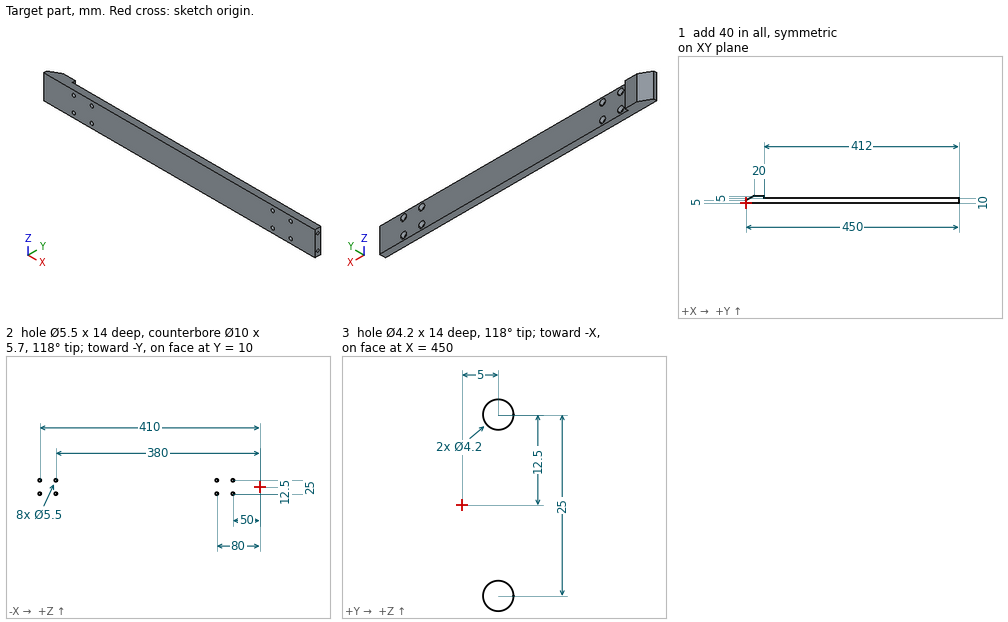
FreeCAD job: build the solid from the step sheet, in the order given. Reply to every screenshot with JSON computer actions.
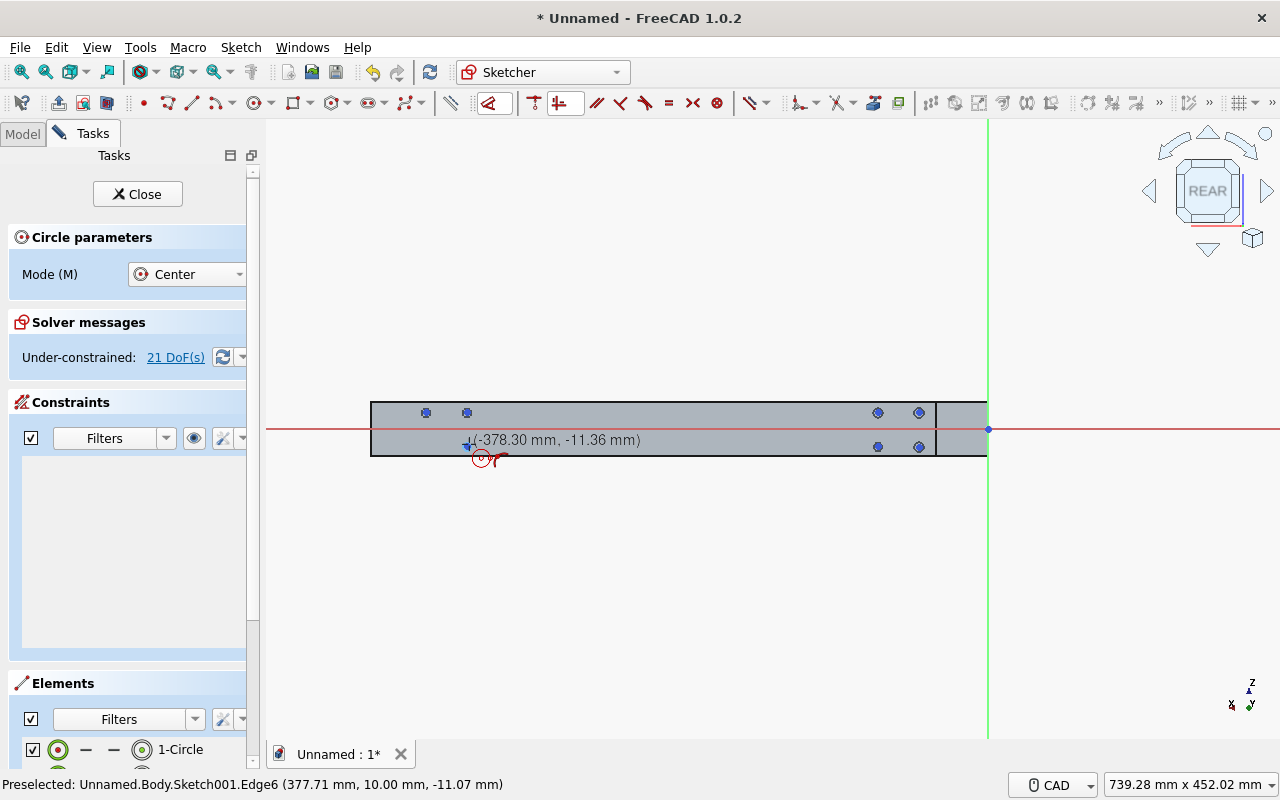
{"action": "scroll", "coordinate": [426, 446], "scroll_direction": "up", "scroll_amount": 9}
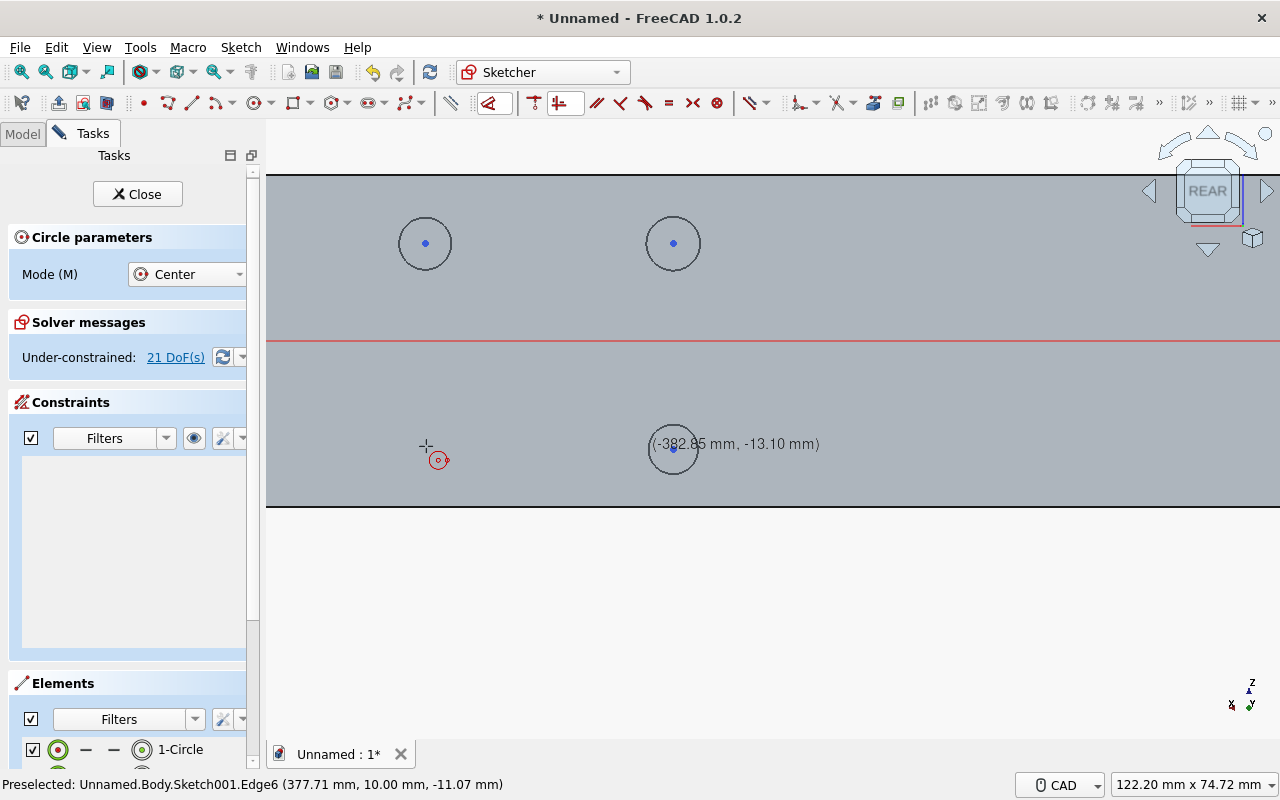
{"action": "scroll", "coordinate": [426, 446], "scroll_direction": "down", "scroll_amount": 9}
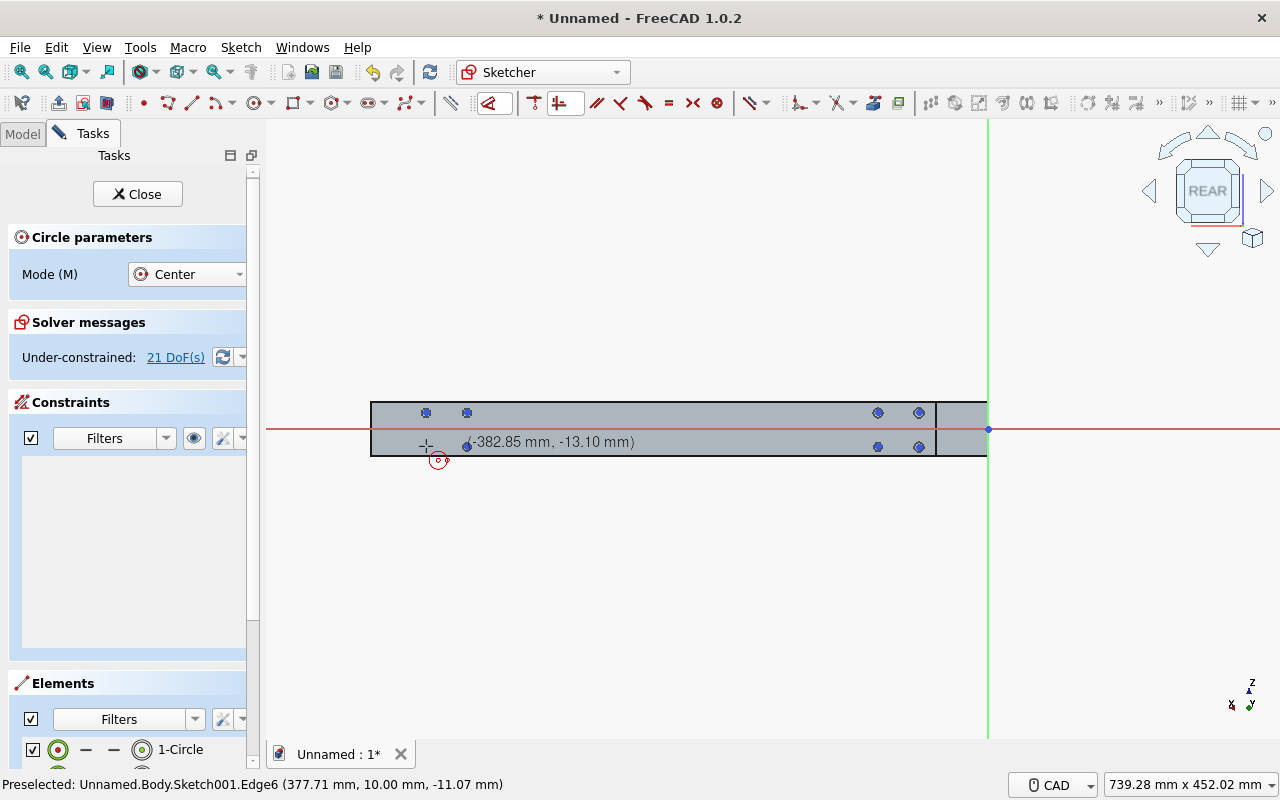
{"action": "left_click", "coordinate": [426, 446]}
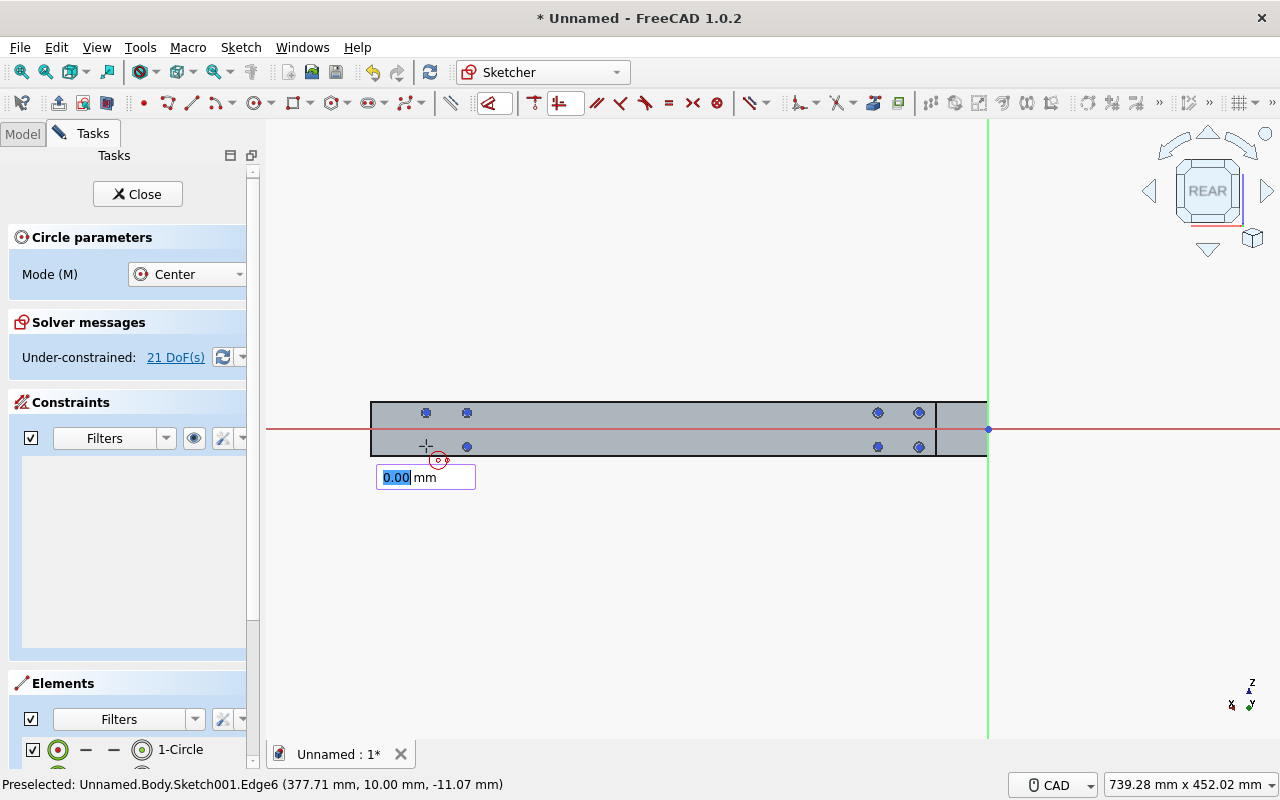
{"action": "scroll", "coordinate": [428, 444], "scroll_direction": "up", "scroll_amount": 8}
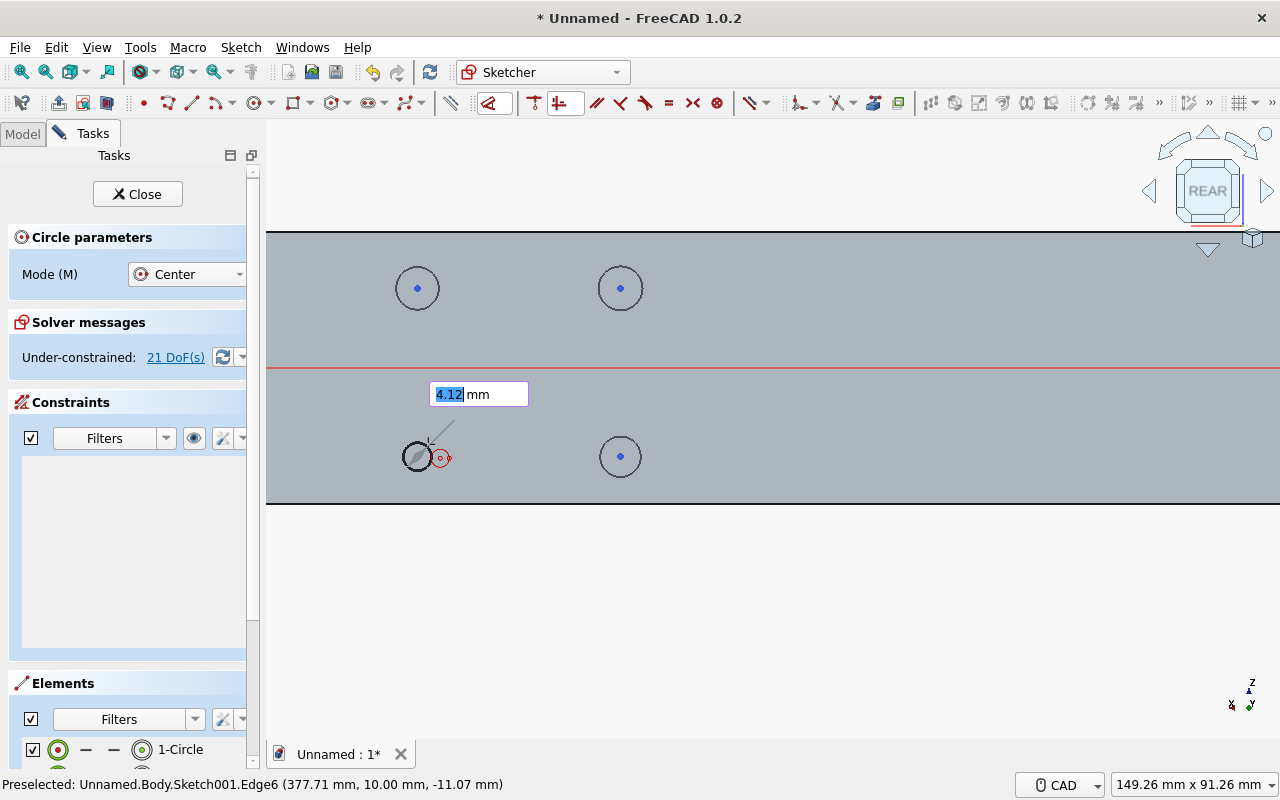
{"action": "left_click", "coordinate": [429, 440]}
{"action": "key", "text": "Escape"}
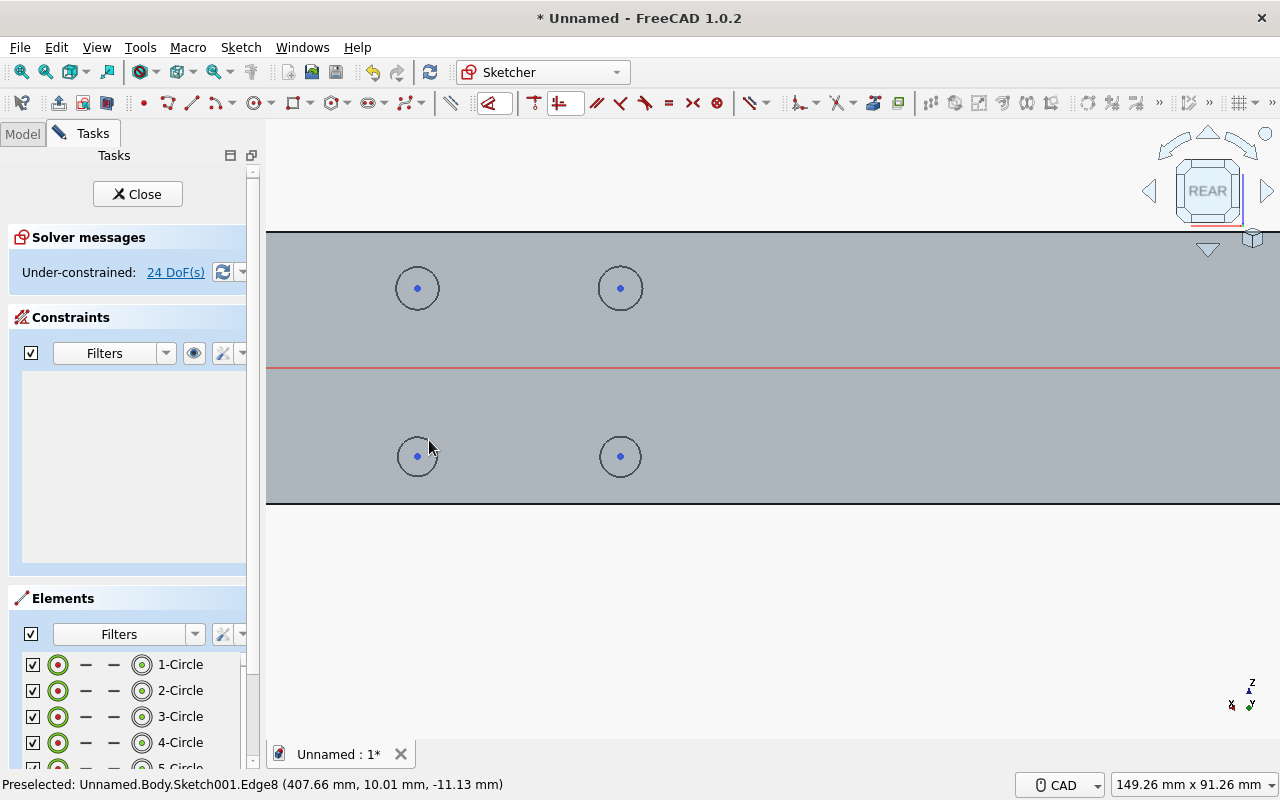
{"action": "scroll", "coordinate": [428, 444], "scroll_direction": "down", "scroll_amount": 8}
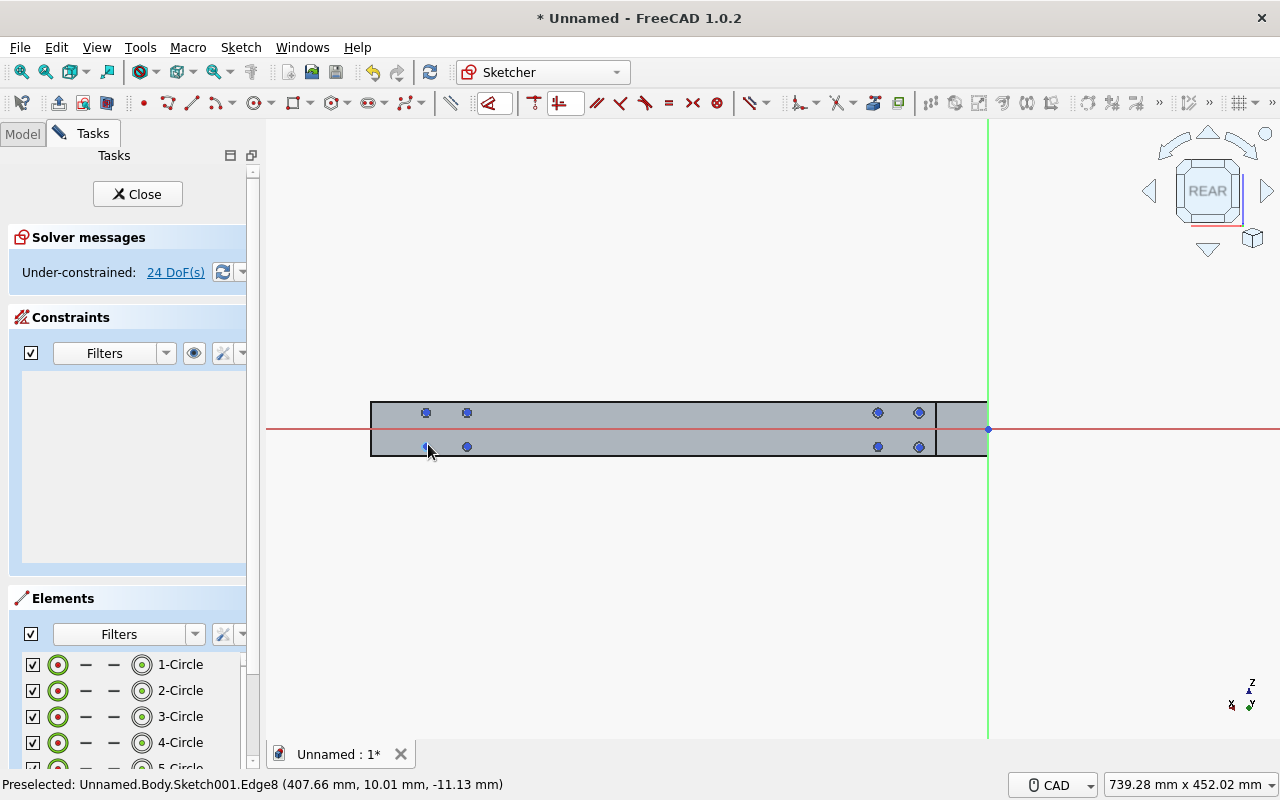
{"action": "scroll", "coordinate": [922, 444], "scroll_direction": "up", "scroll_amount": 6}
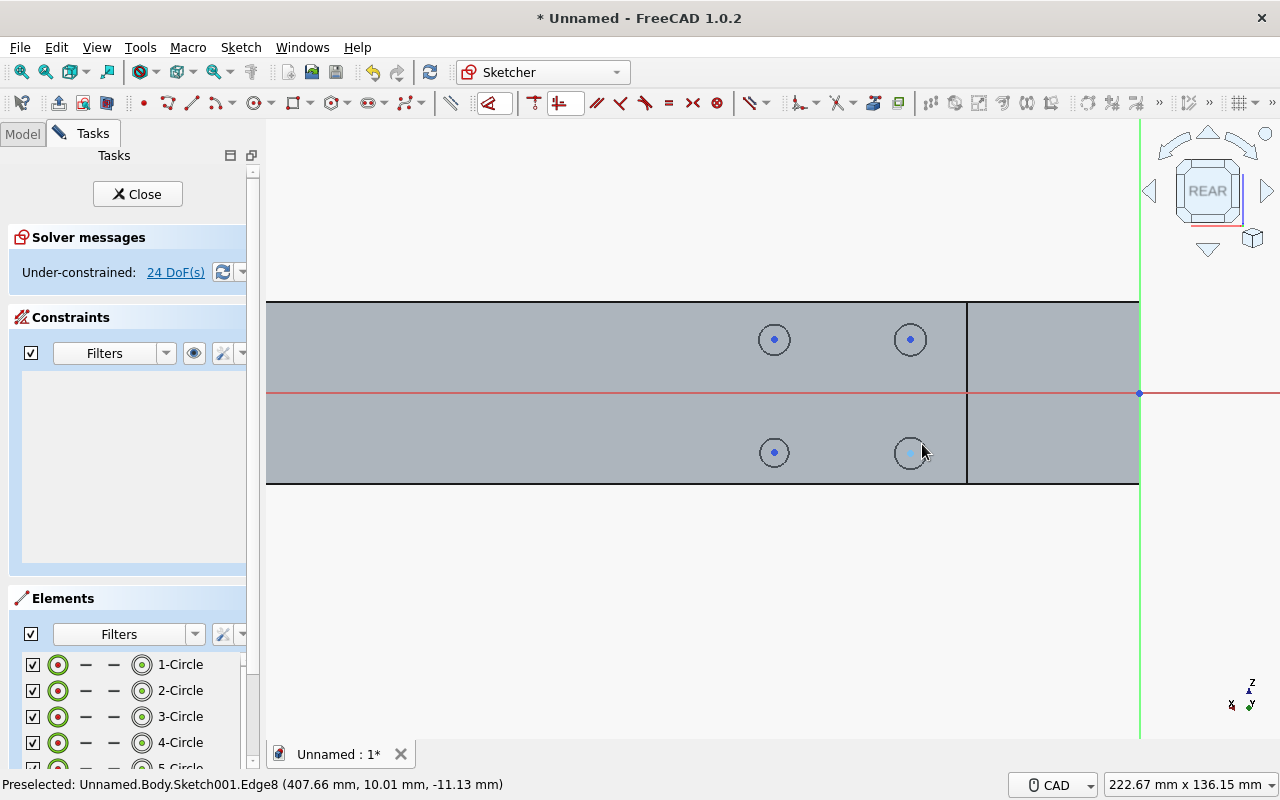
{"action": "left_click", "coordinate": [922, 442]}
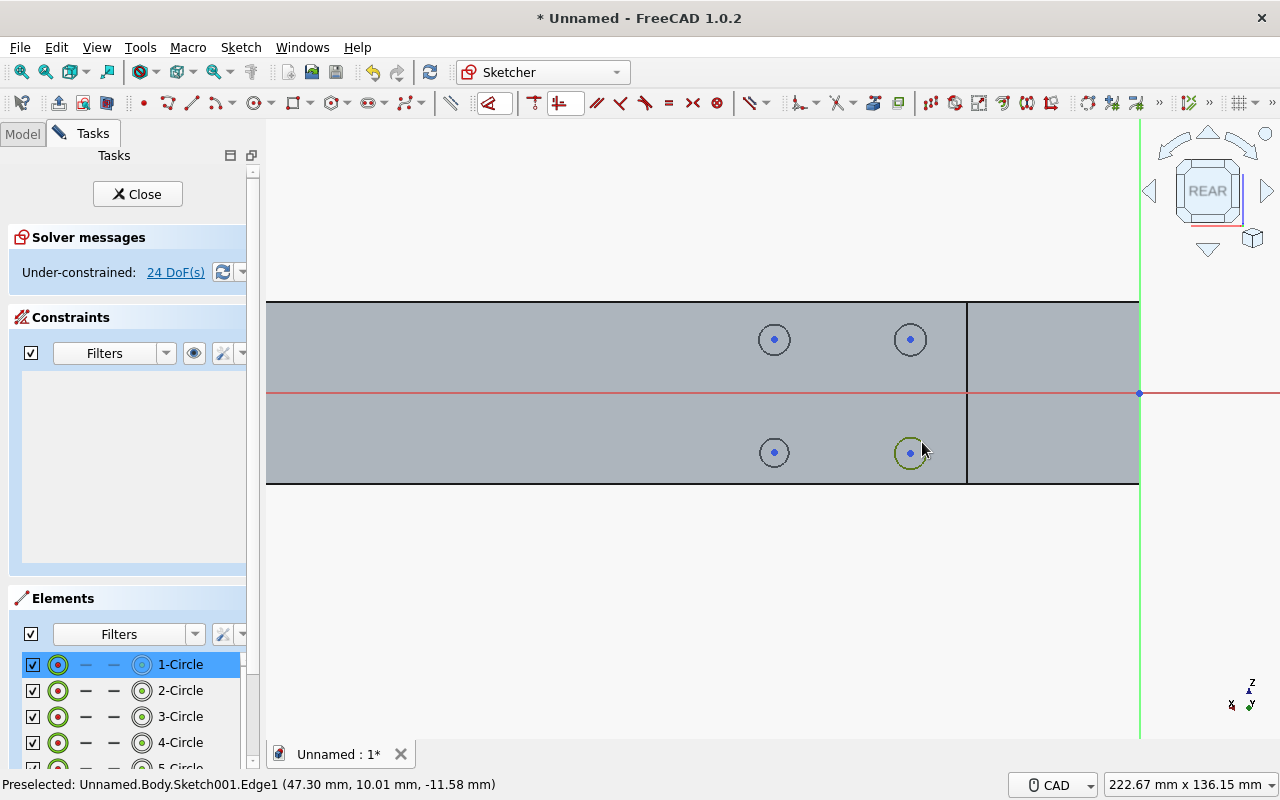
{"action": "left_click", "coordinate": [784, 443]}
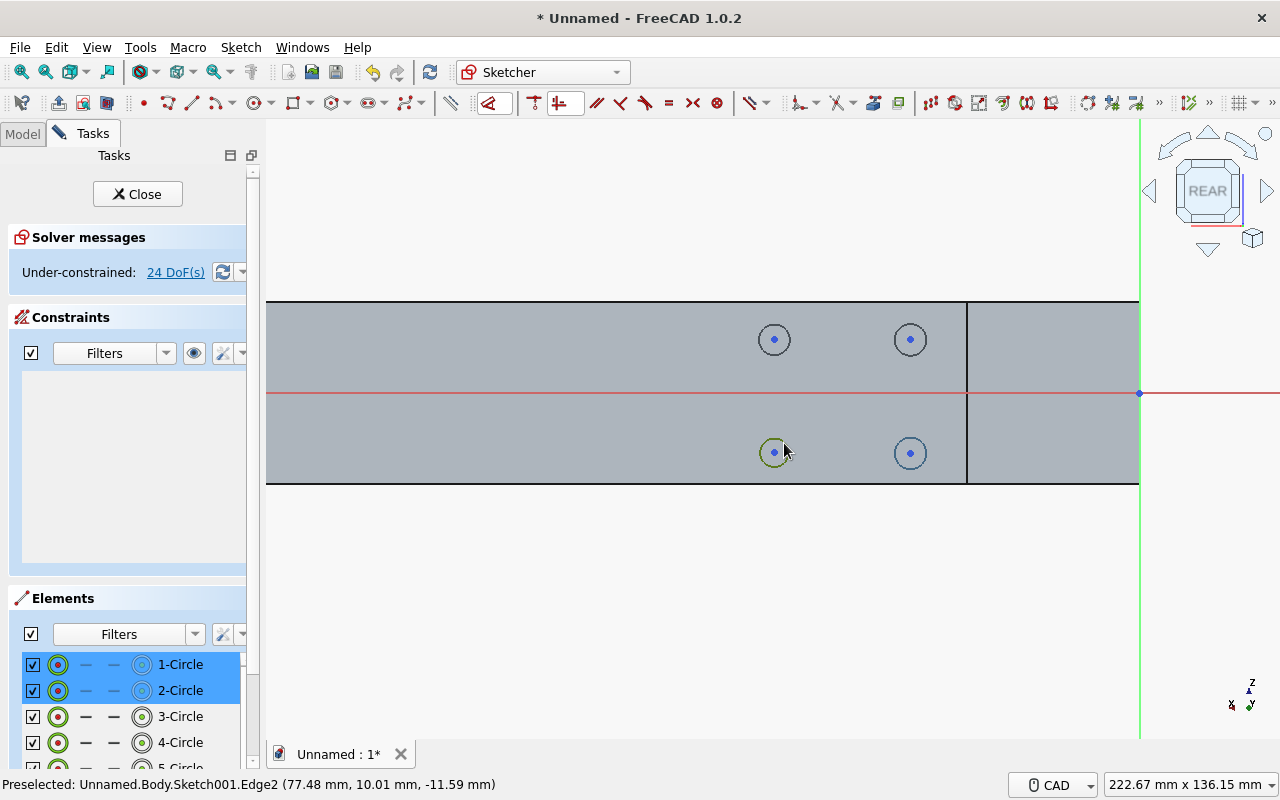
{"action": "left_click", "coordinate": [922, 329]}